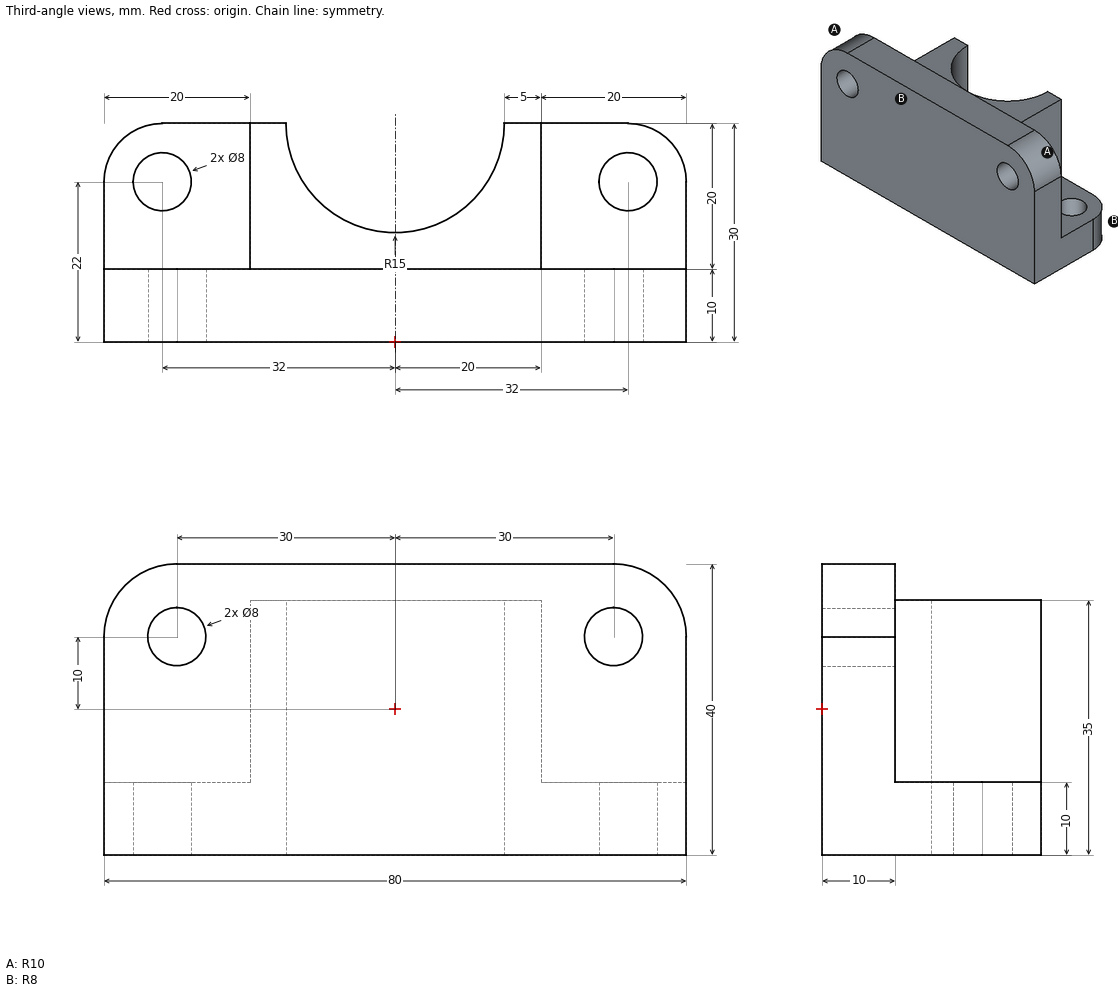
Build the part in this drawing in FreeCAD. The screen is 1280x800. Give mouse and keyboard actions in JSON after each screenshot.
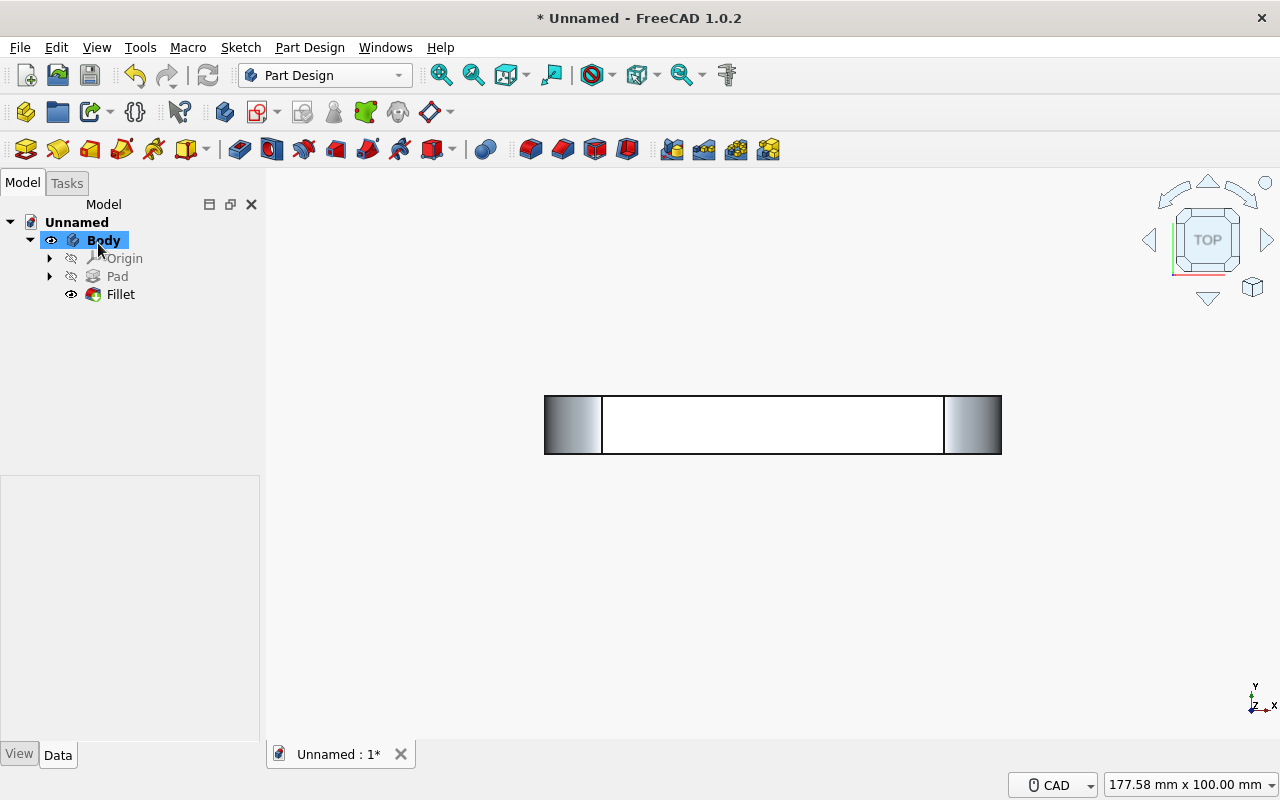
{"action": "left_click", "coordinate": [442, 76]}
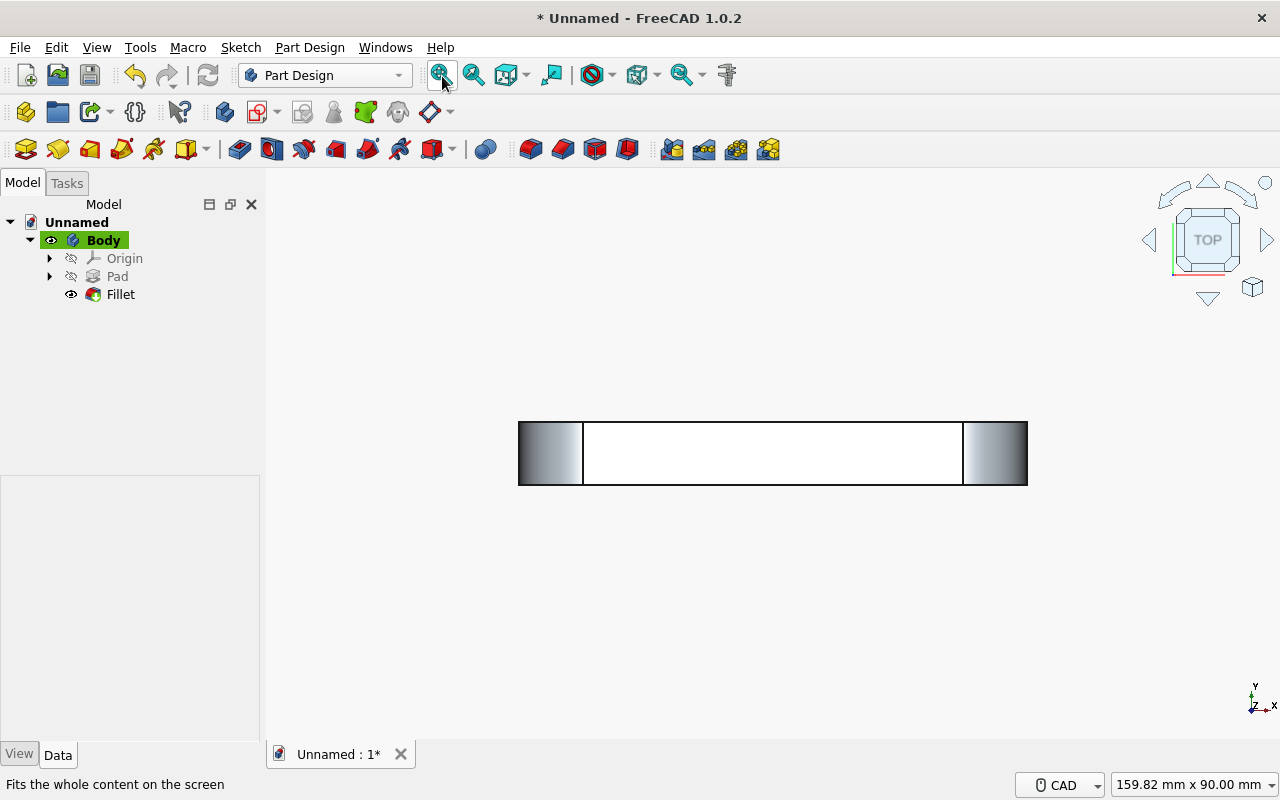
{"action": "key", "text": "5"}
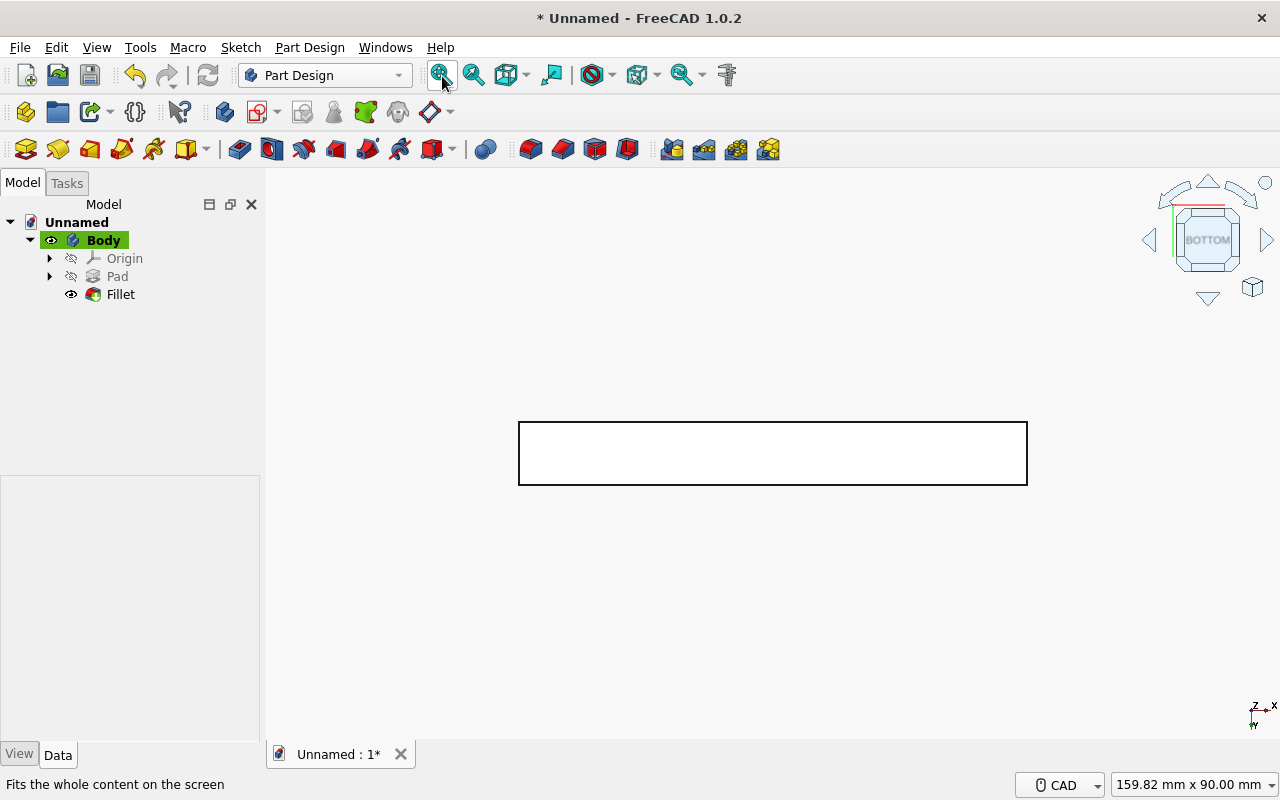
{"action": "left_click", "coordinate": [991, 452]}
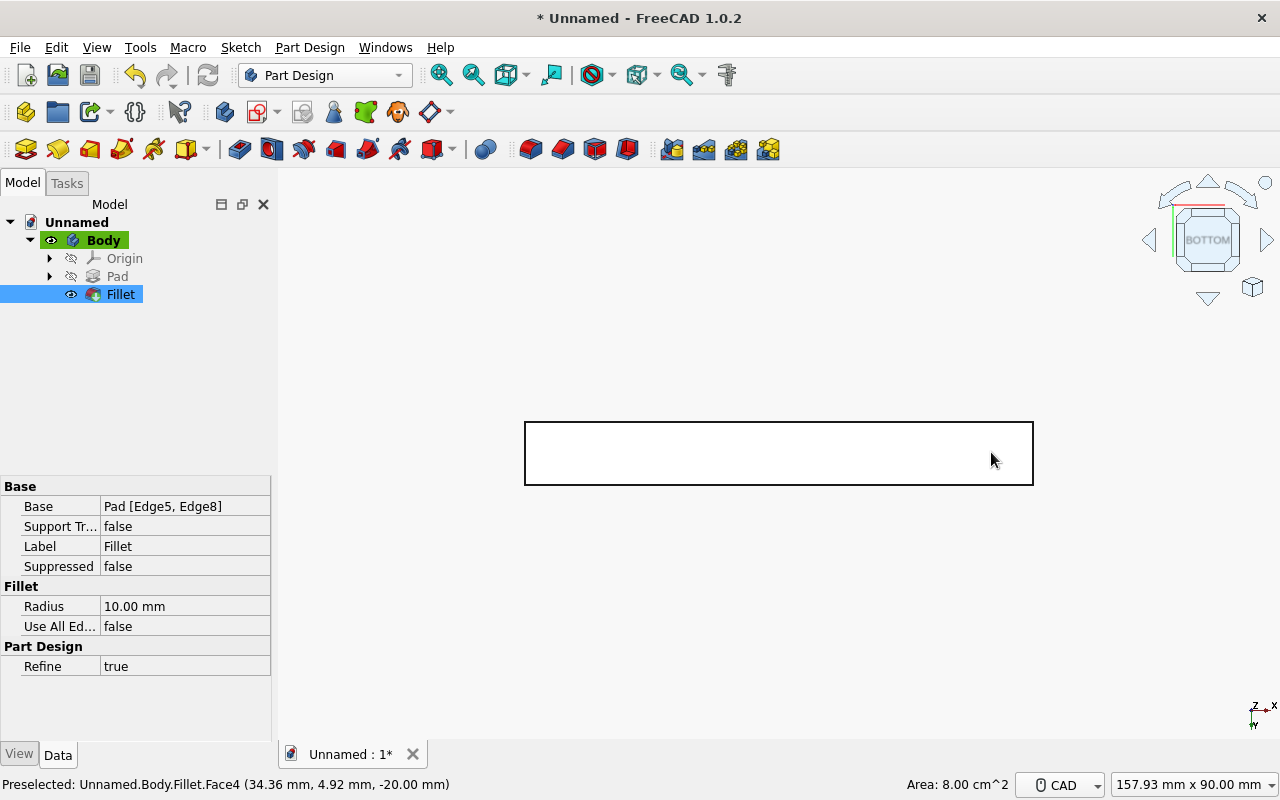
{"action": "left_click", "coordinate": [258, 112]}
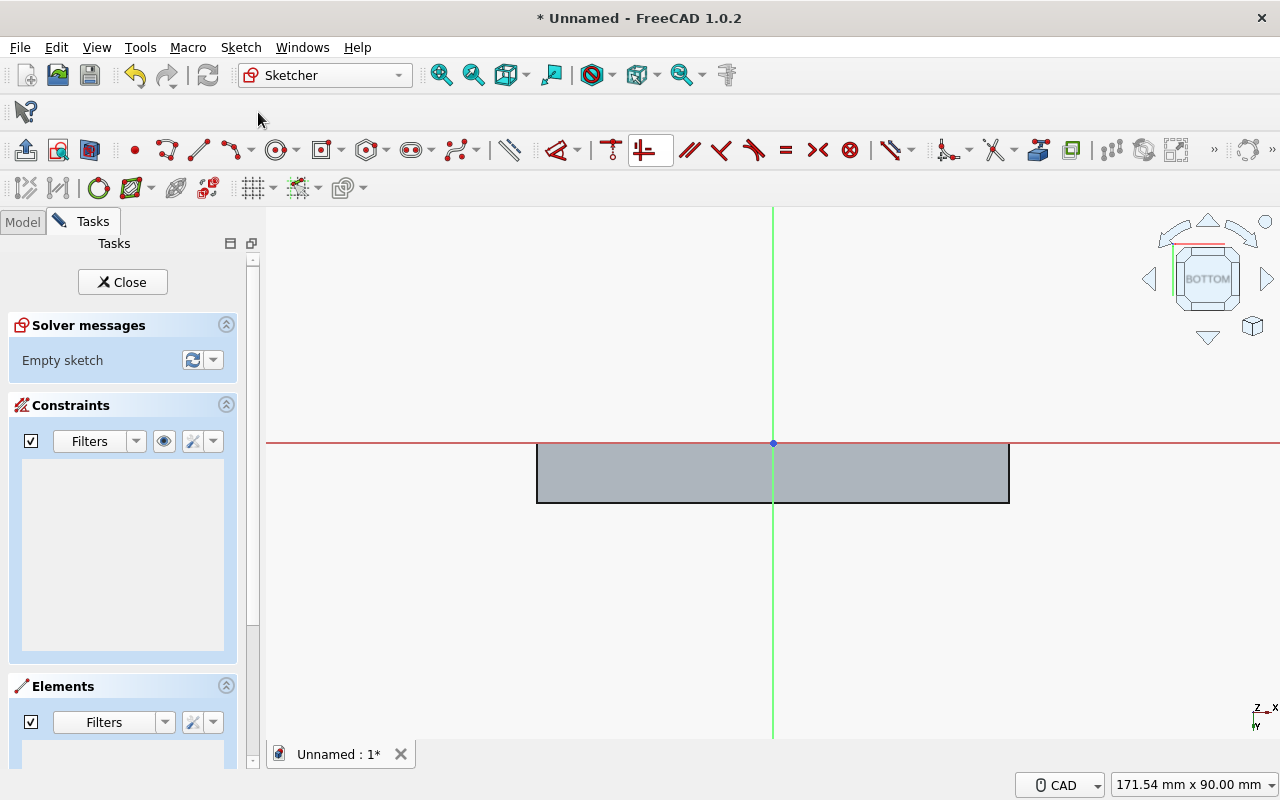
{"action": "scroll", "coordinate": [856, 604], "scroll_direction": "up", "scroll_amount": 3}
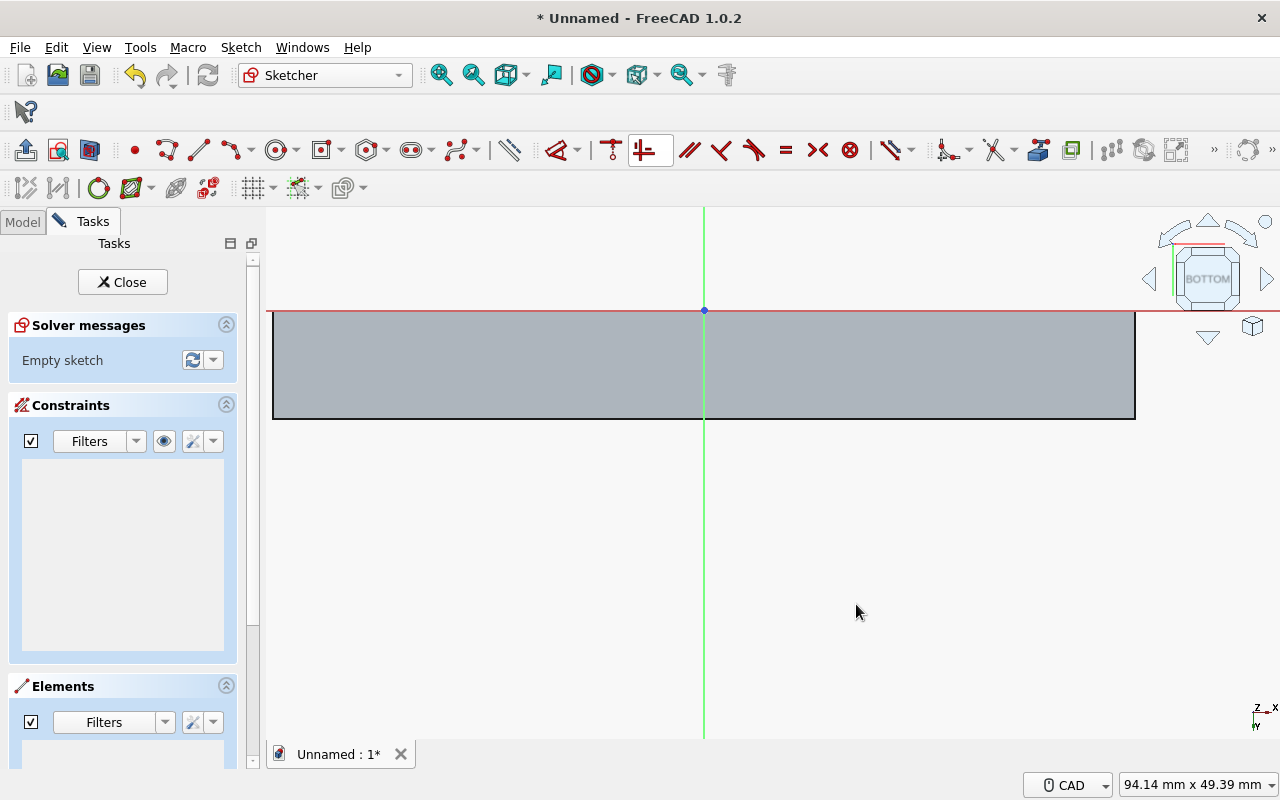
{"action": "left_click", "coordinate": [168, 150]}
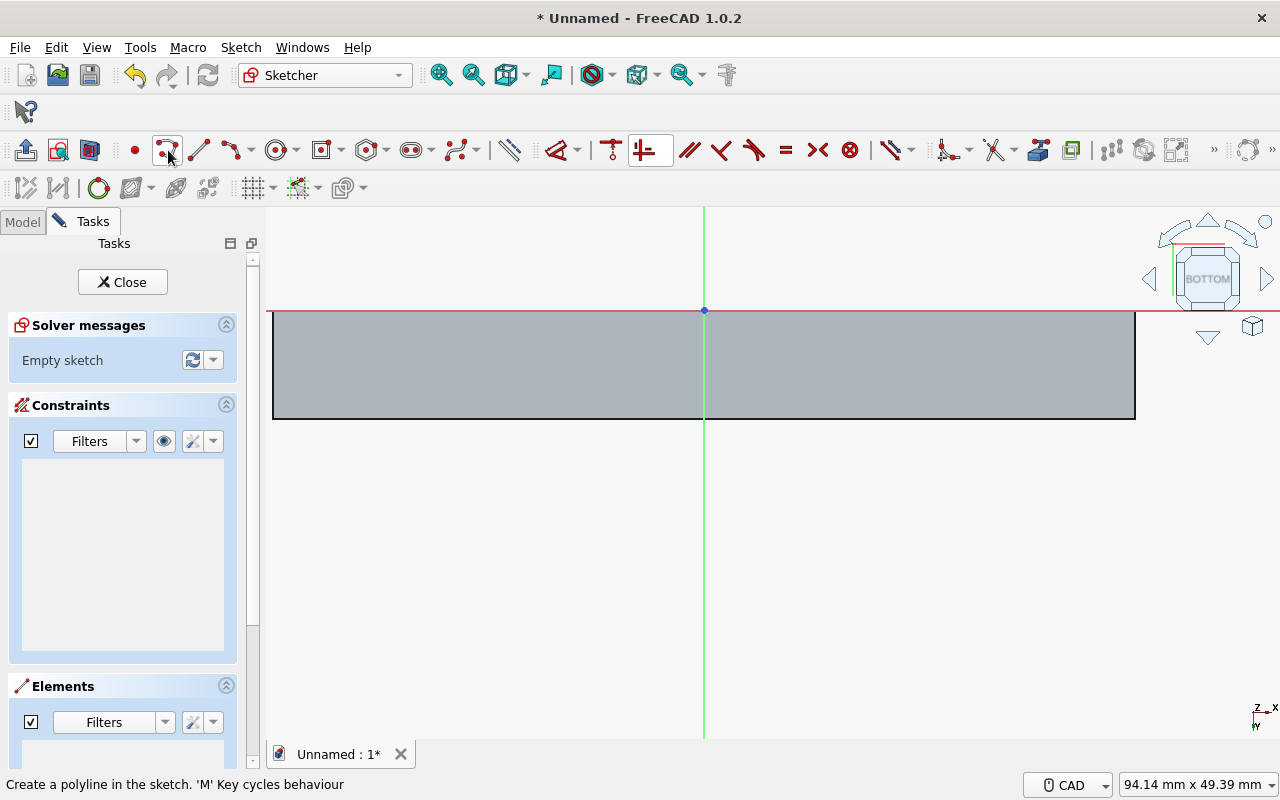
{"action": "left_click", "coordinate": [866, 634]}
{"action": "left_click", "coordinate": [920, 634]}
{"action": "left_click", "coordinate": [920, 419]}
{"action": "left_click", "coordinate": [489, 419]}
{"action": "left_click", "coordinate": [489, 634]}
{"action": "left_click", "coordinate": [543, 634]}
{"action": "right_click", "coordinate": [543, 634]}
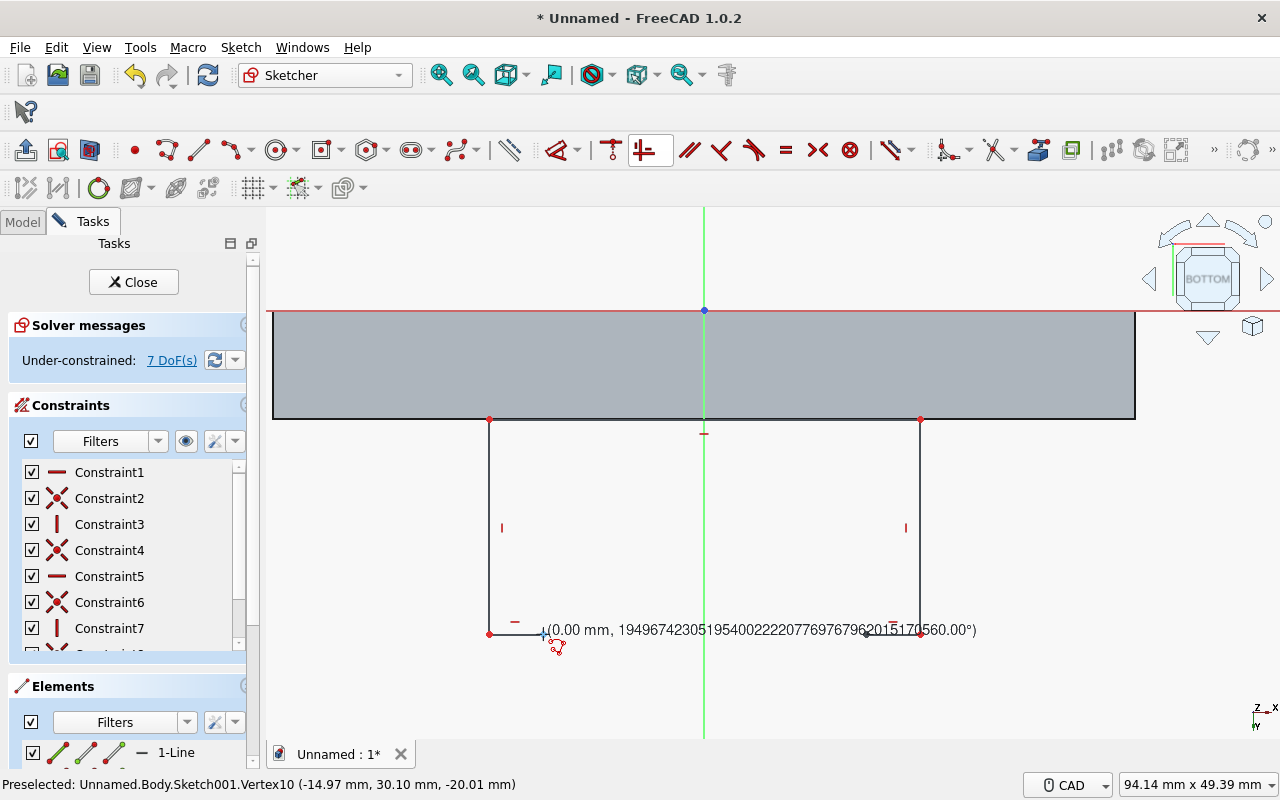
{"action": "left_click", "coordinate": [232, 150]}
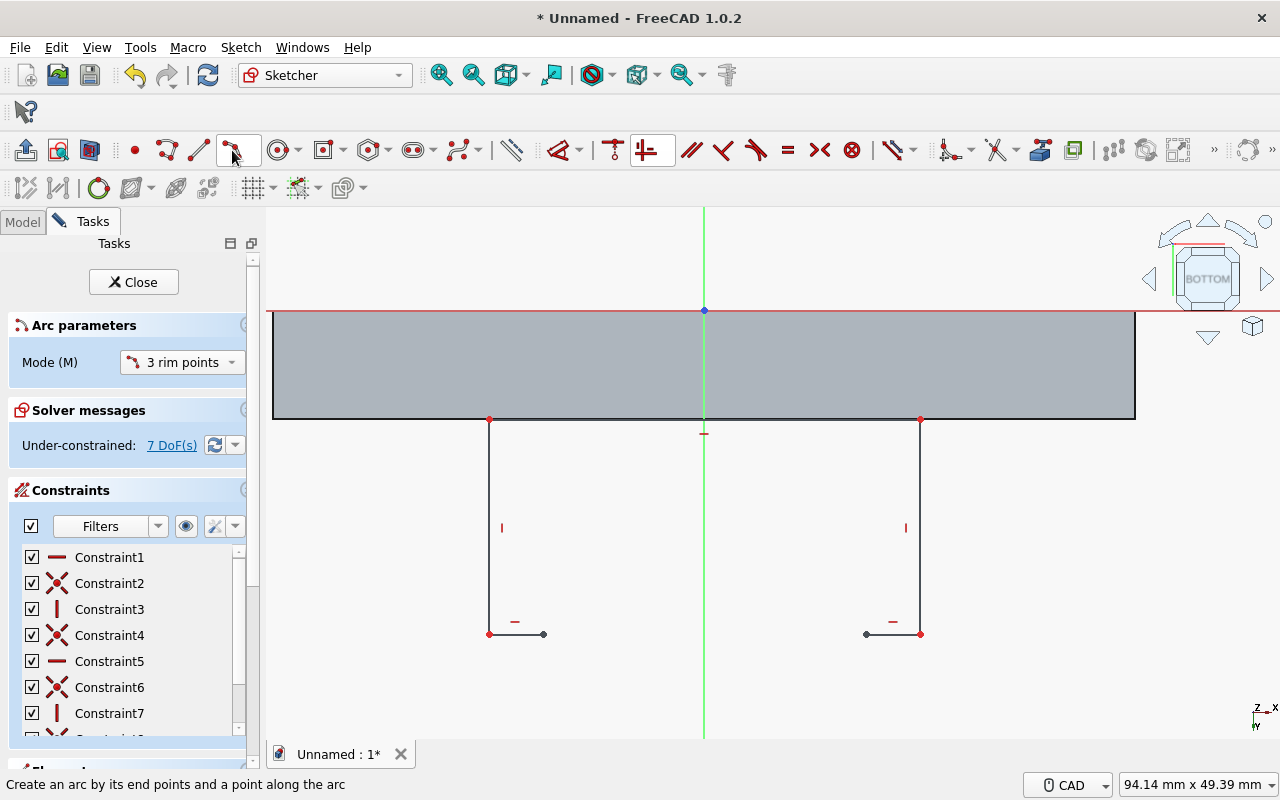
{"action": "left_click", "coordinate": [543, 635]}
{"action": "left_click", "coordinate": [866, 635]}
{"action": "left_click", "coordinate": [754, 480]}
{"action": "key", "text": "Escape"}